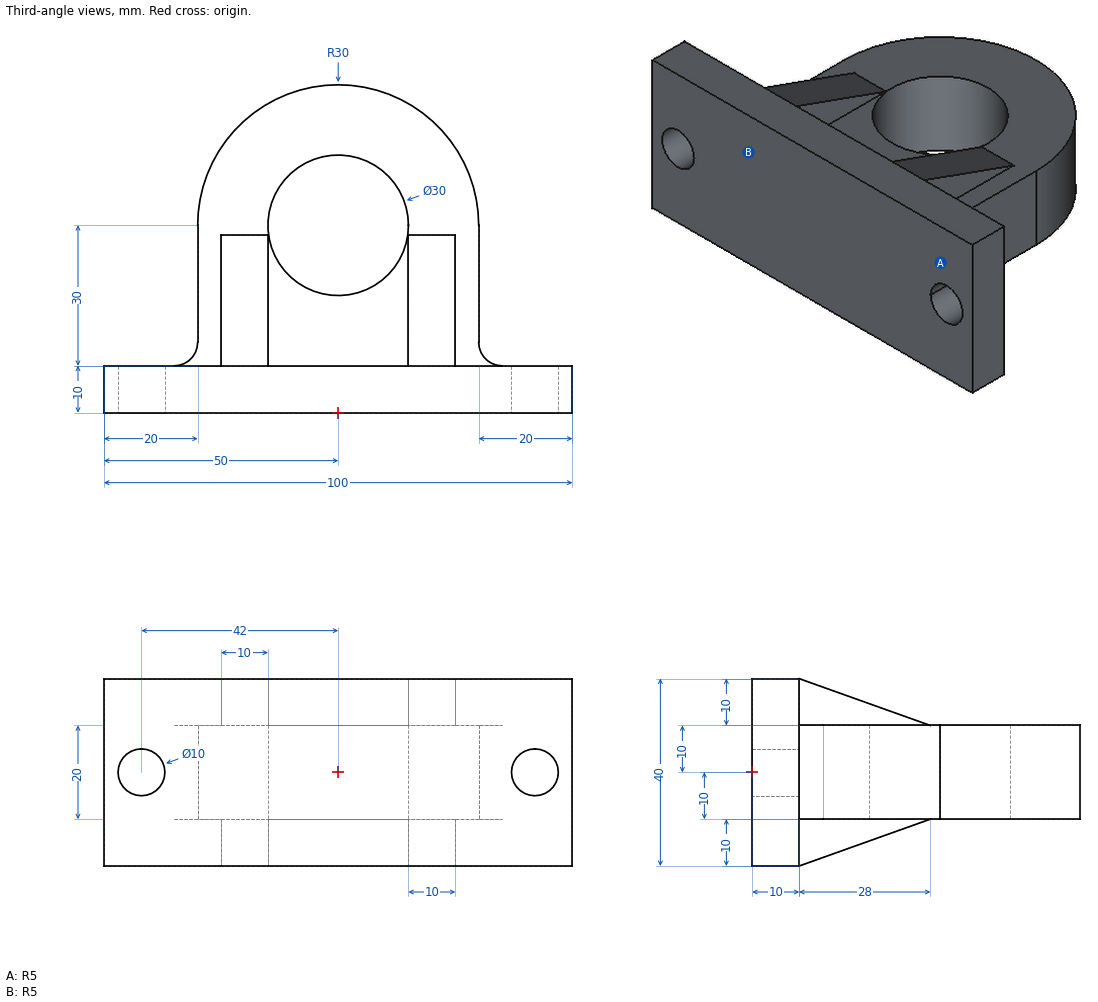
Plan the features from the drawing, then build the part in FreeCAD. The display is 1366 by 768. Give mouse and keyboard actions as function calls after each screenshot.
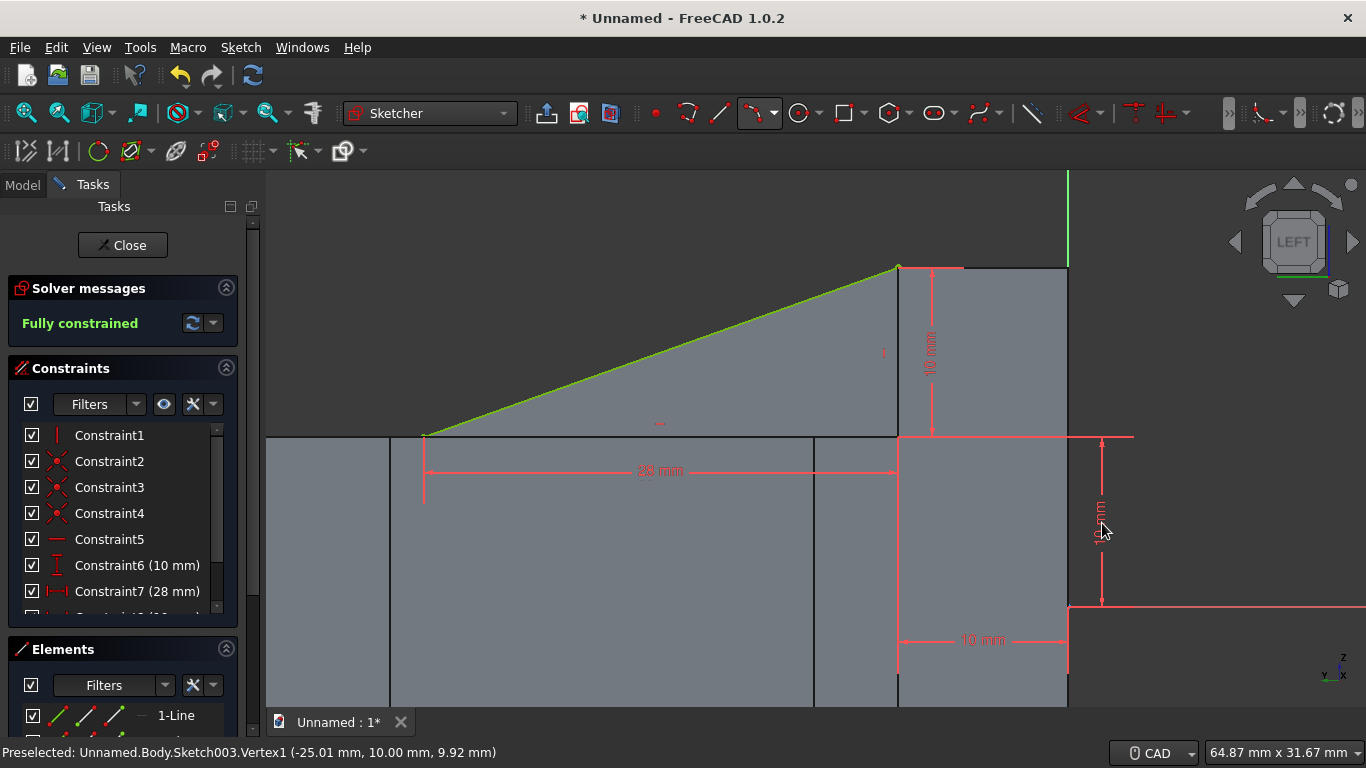
click(123, 245)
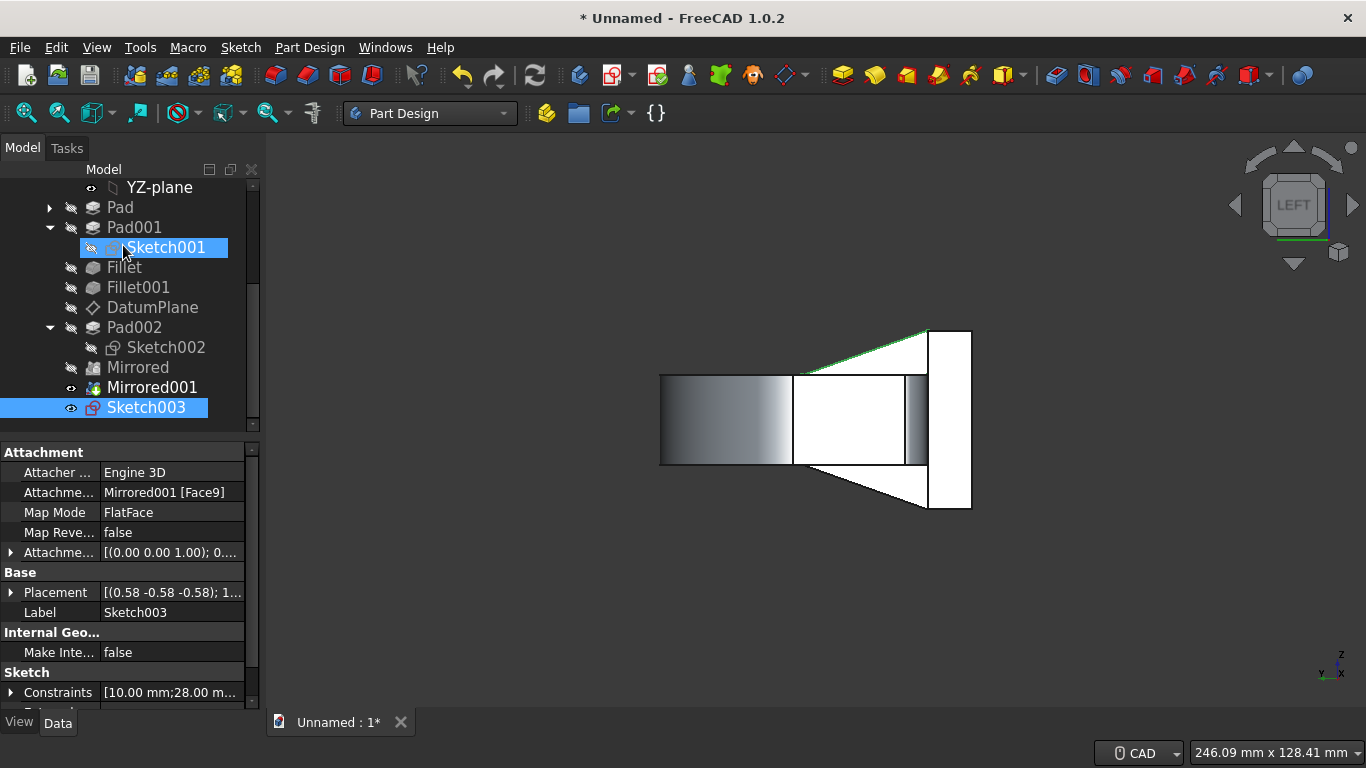
click(844, 76)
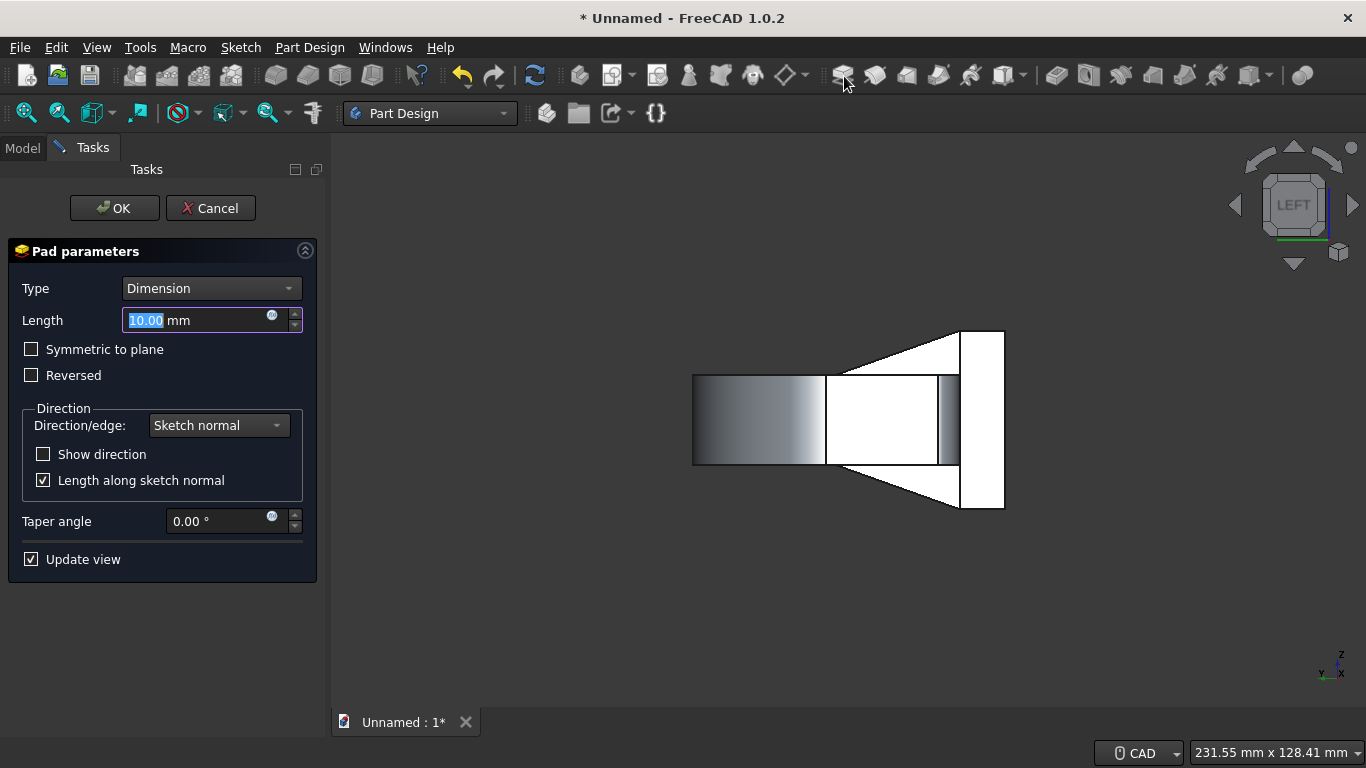
text(10)
key(Tab)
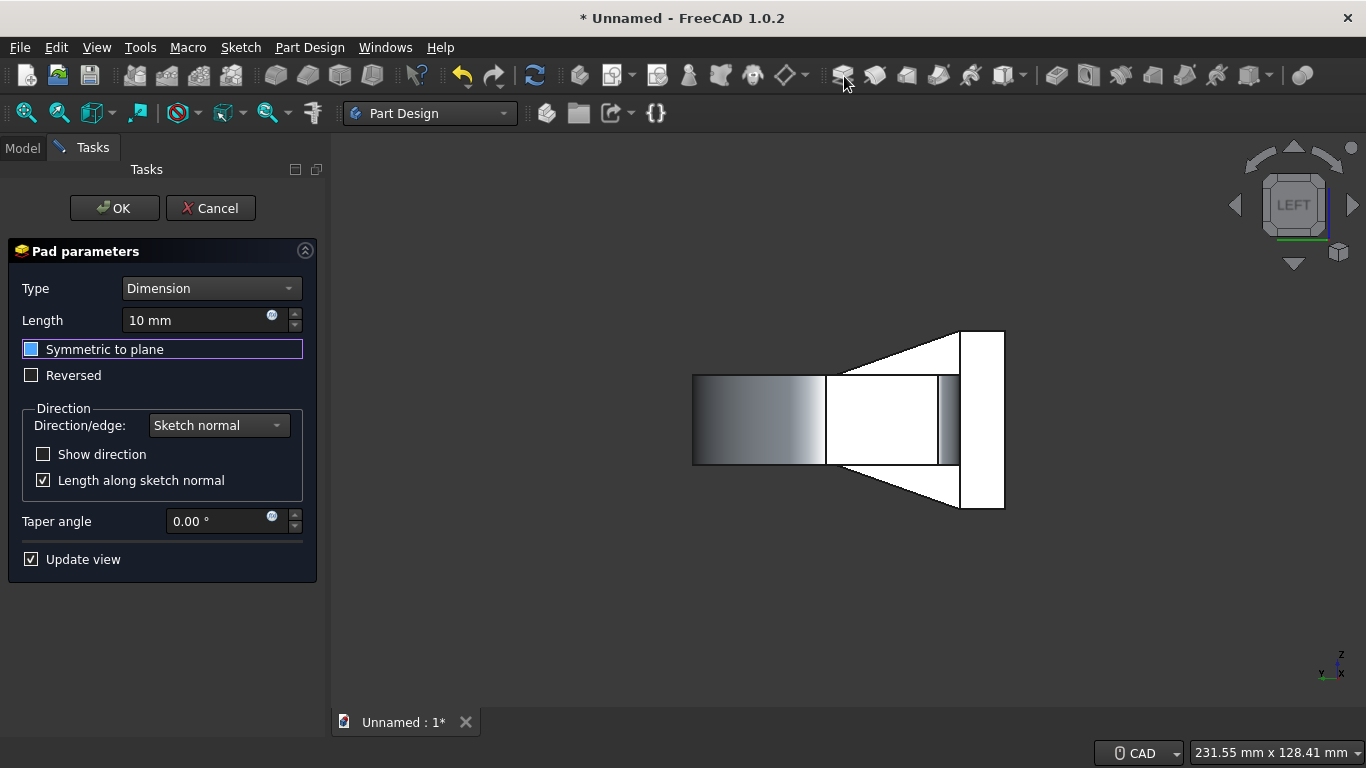
click(30, 375)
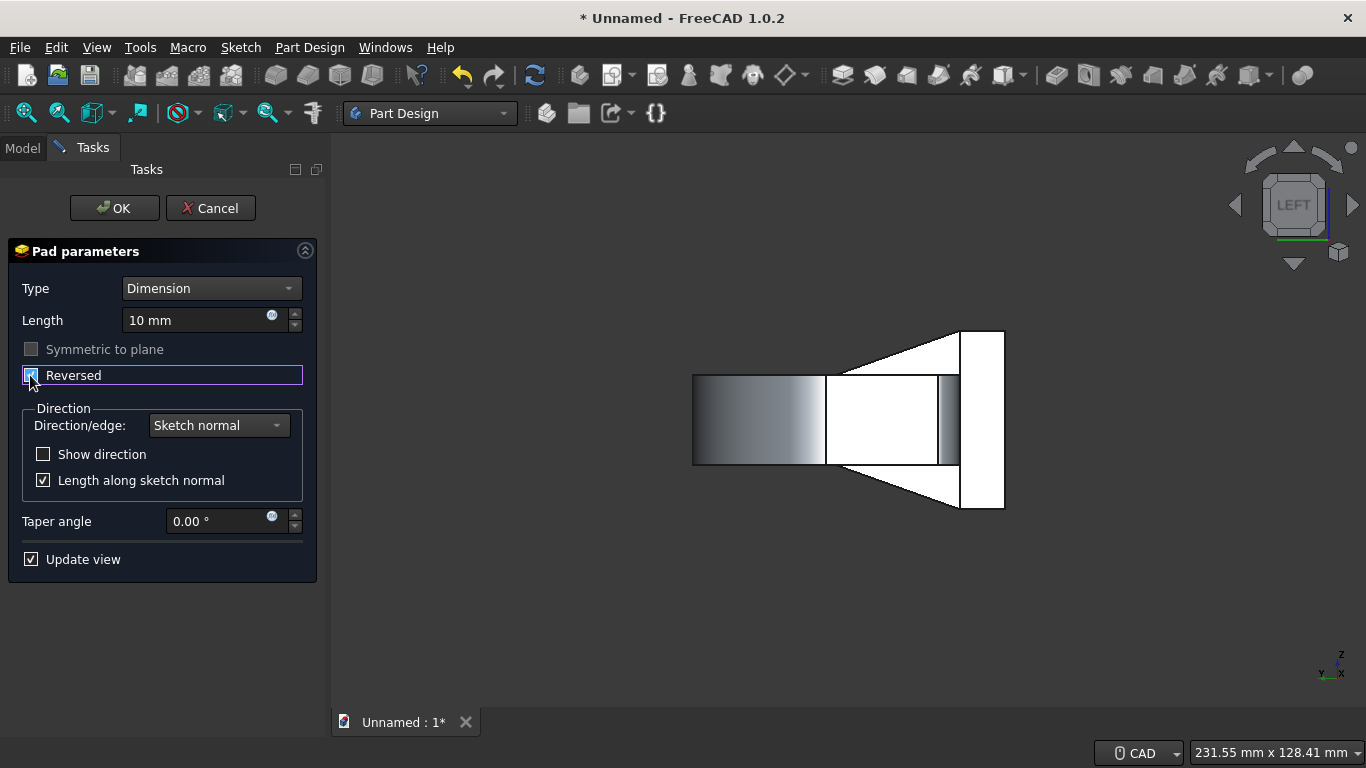
click(115, 208)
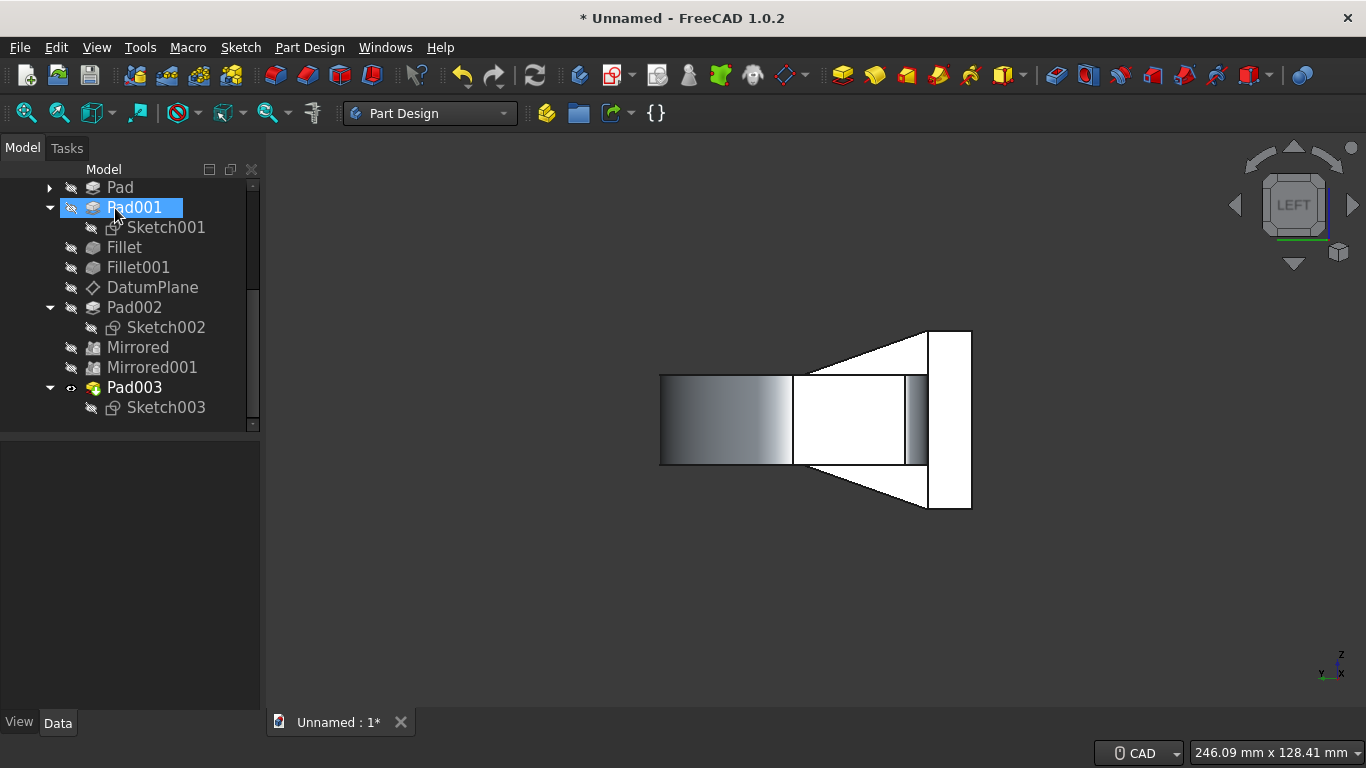
click(28, 114)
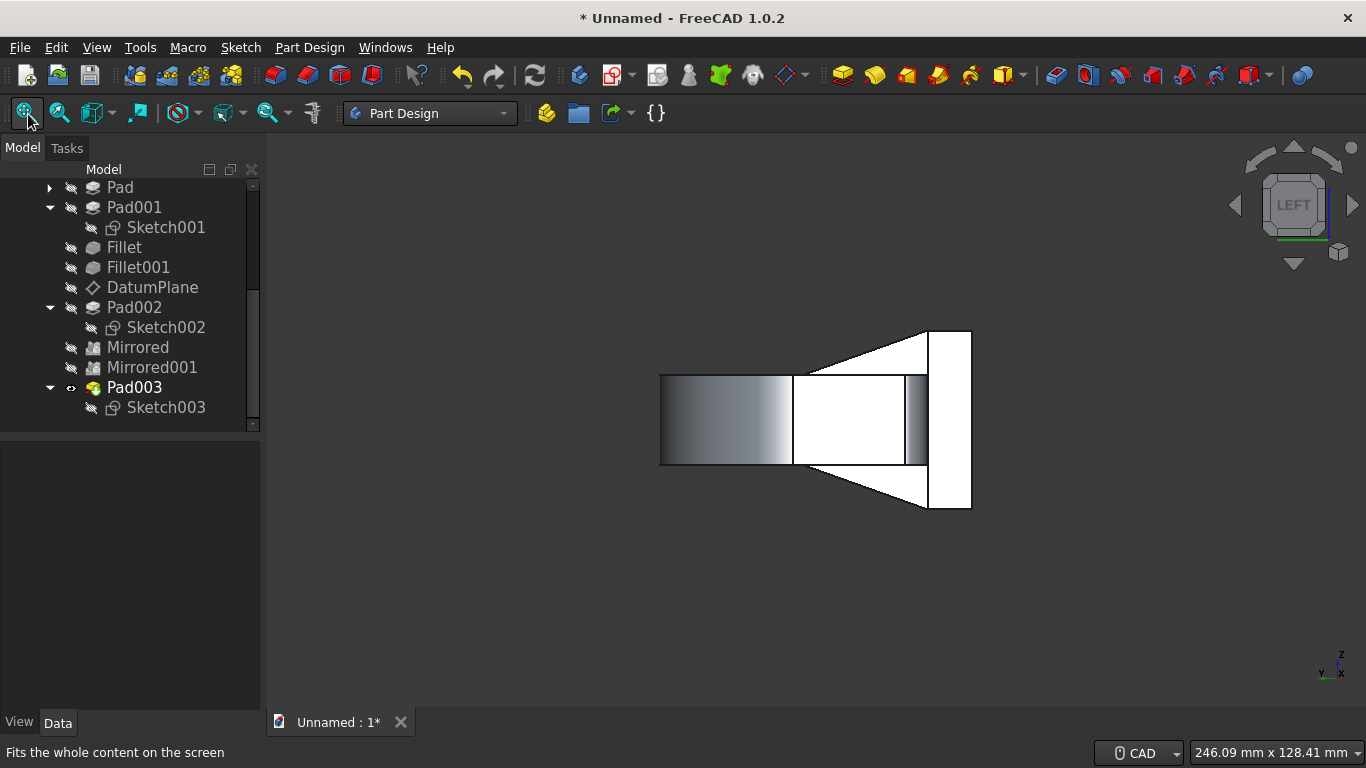
click(612, 76)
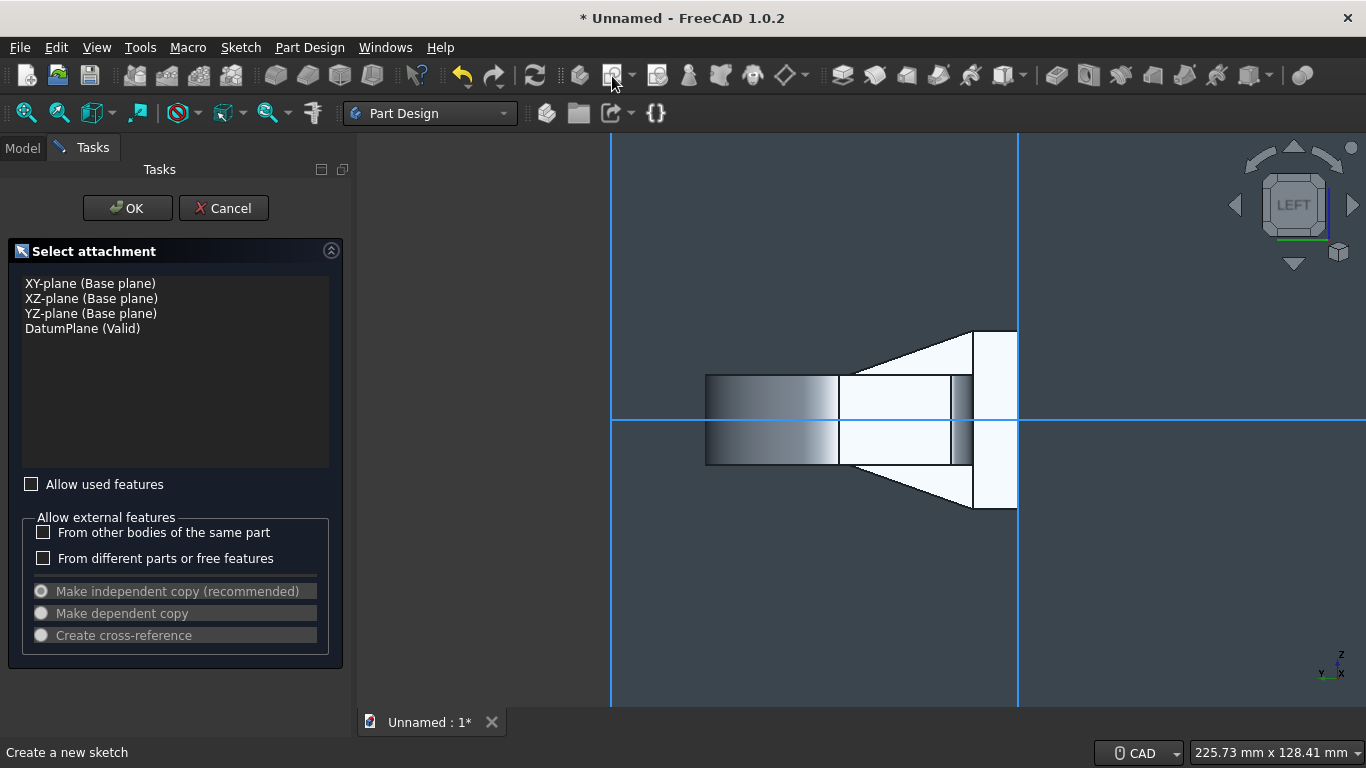
click(82, 298)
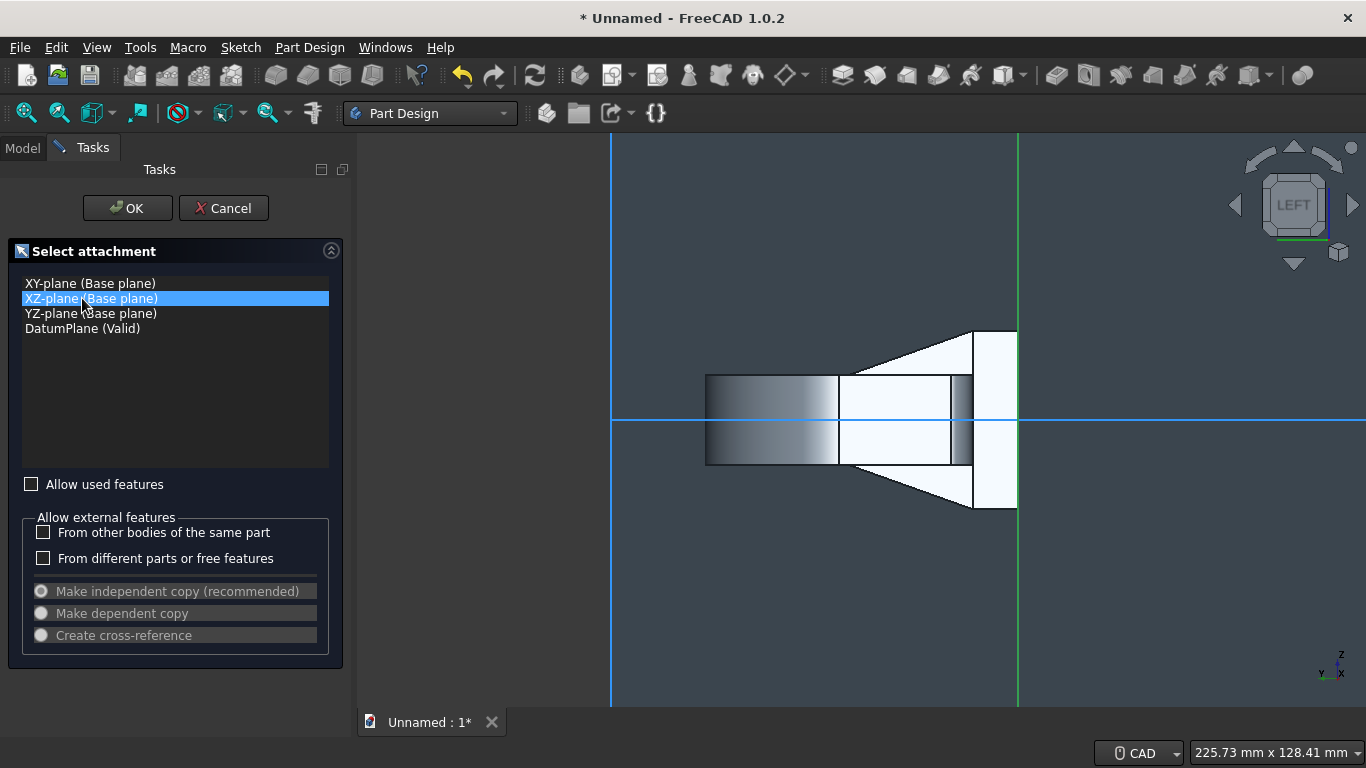
click(128, 208)